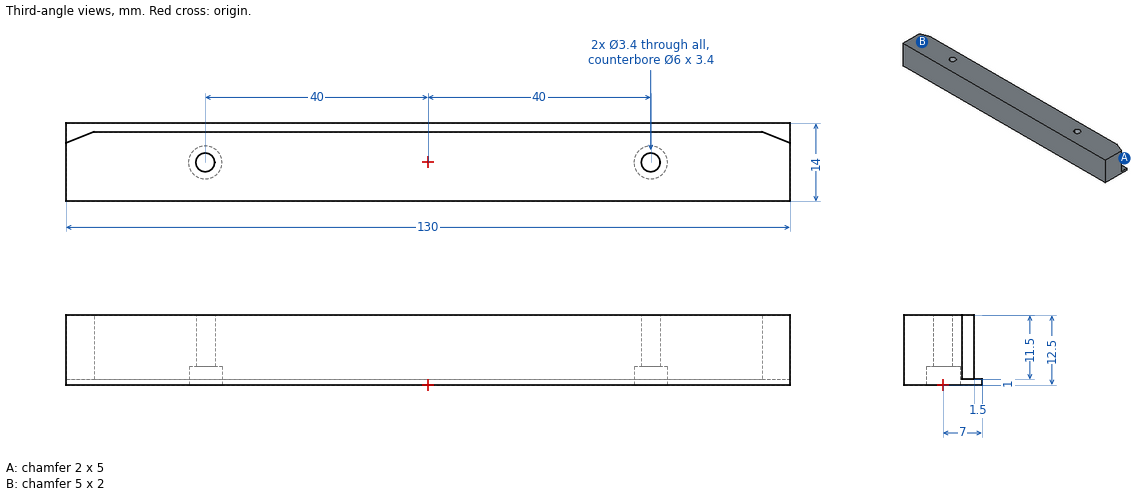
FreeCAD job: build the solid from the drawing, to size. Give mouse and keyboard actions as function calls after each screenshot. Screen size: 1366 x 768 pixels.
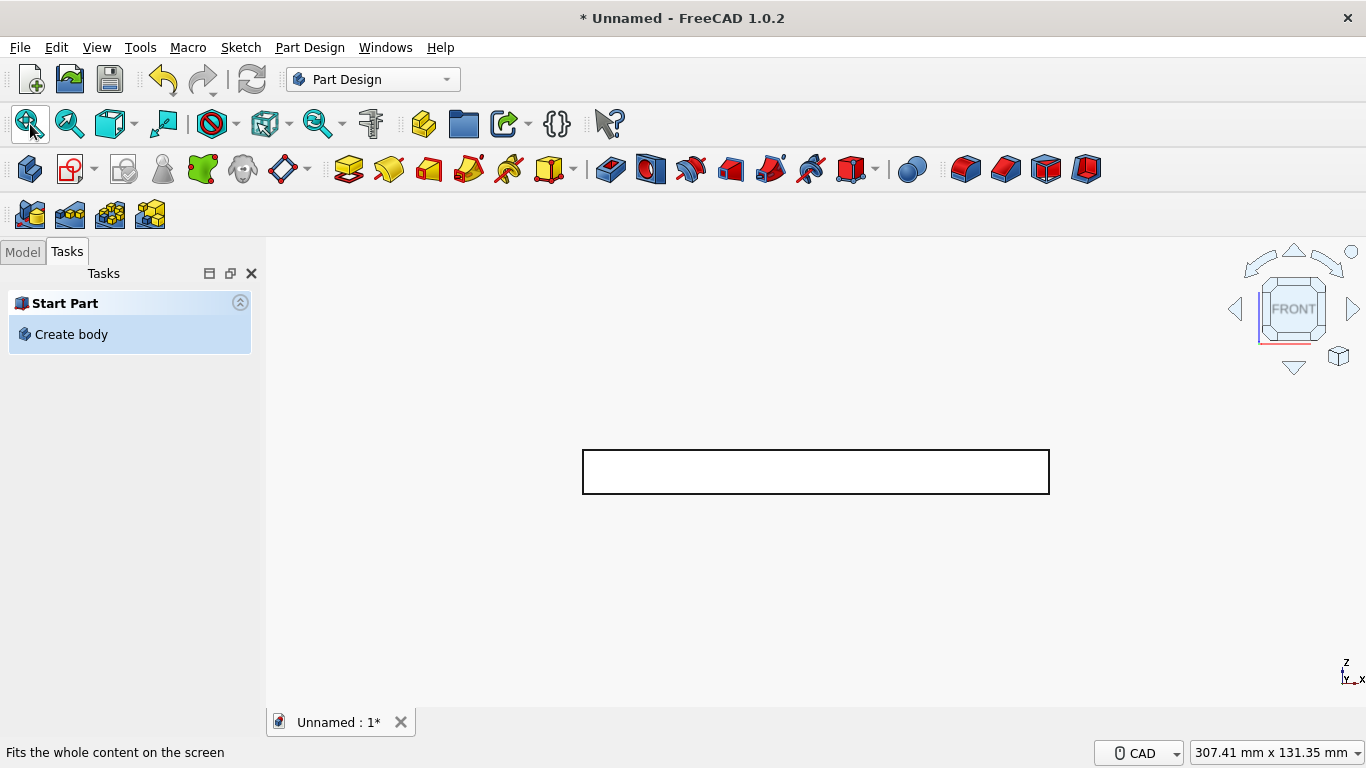
key(3)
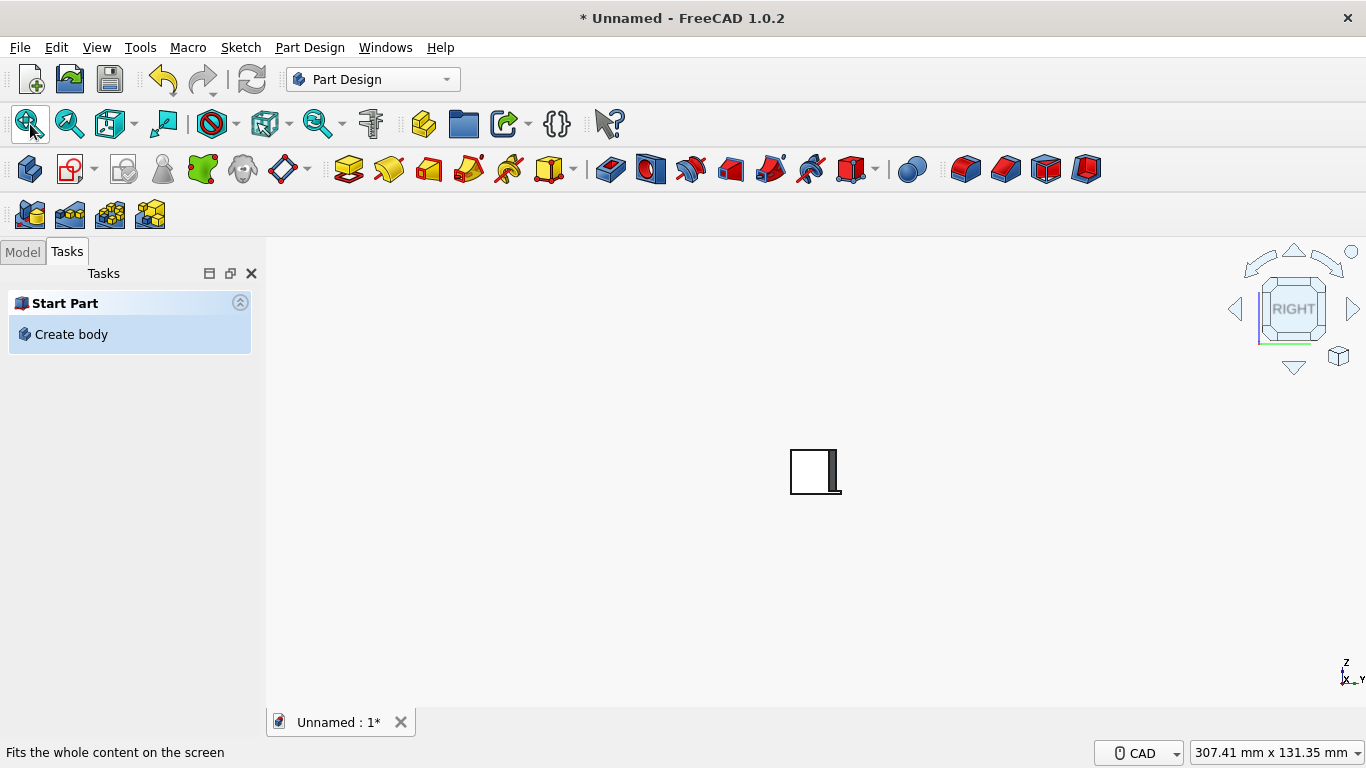
click(30, 124)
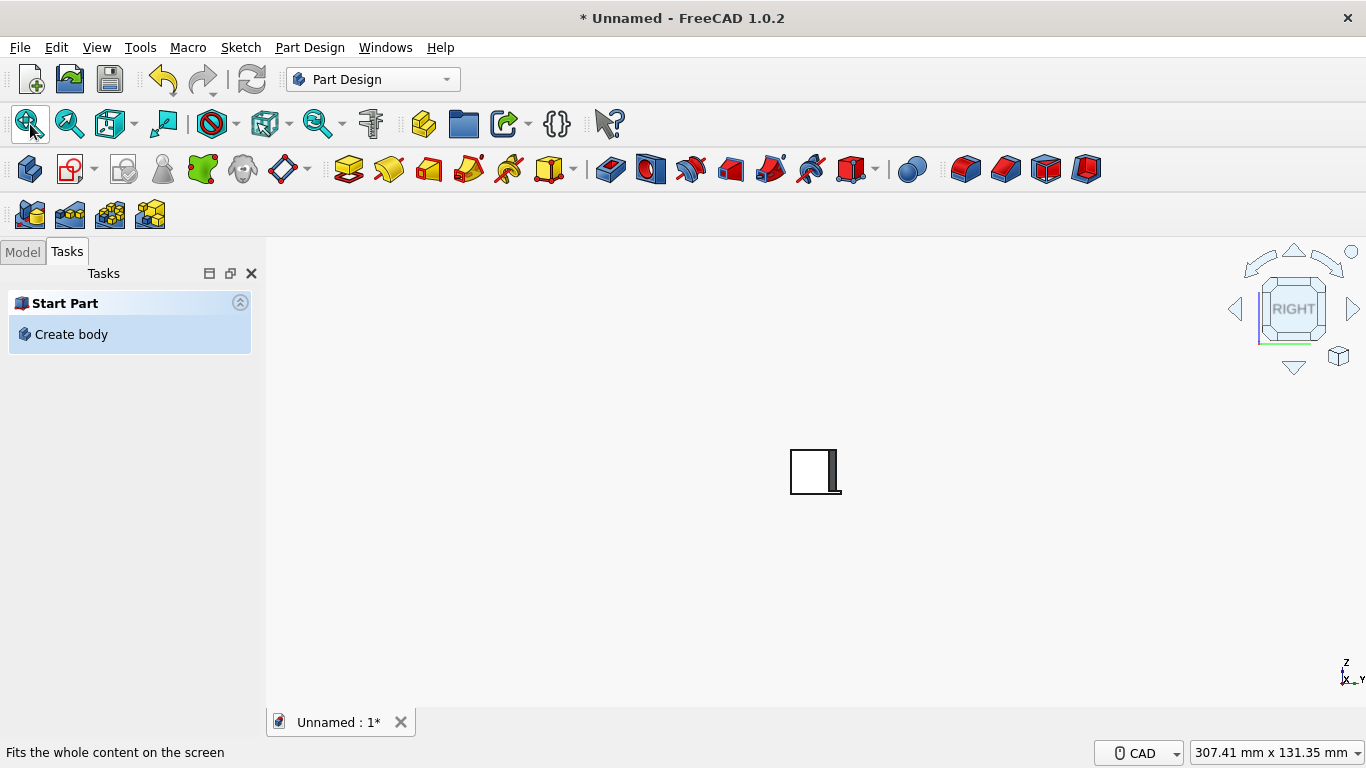
key(5)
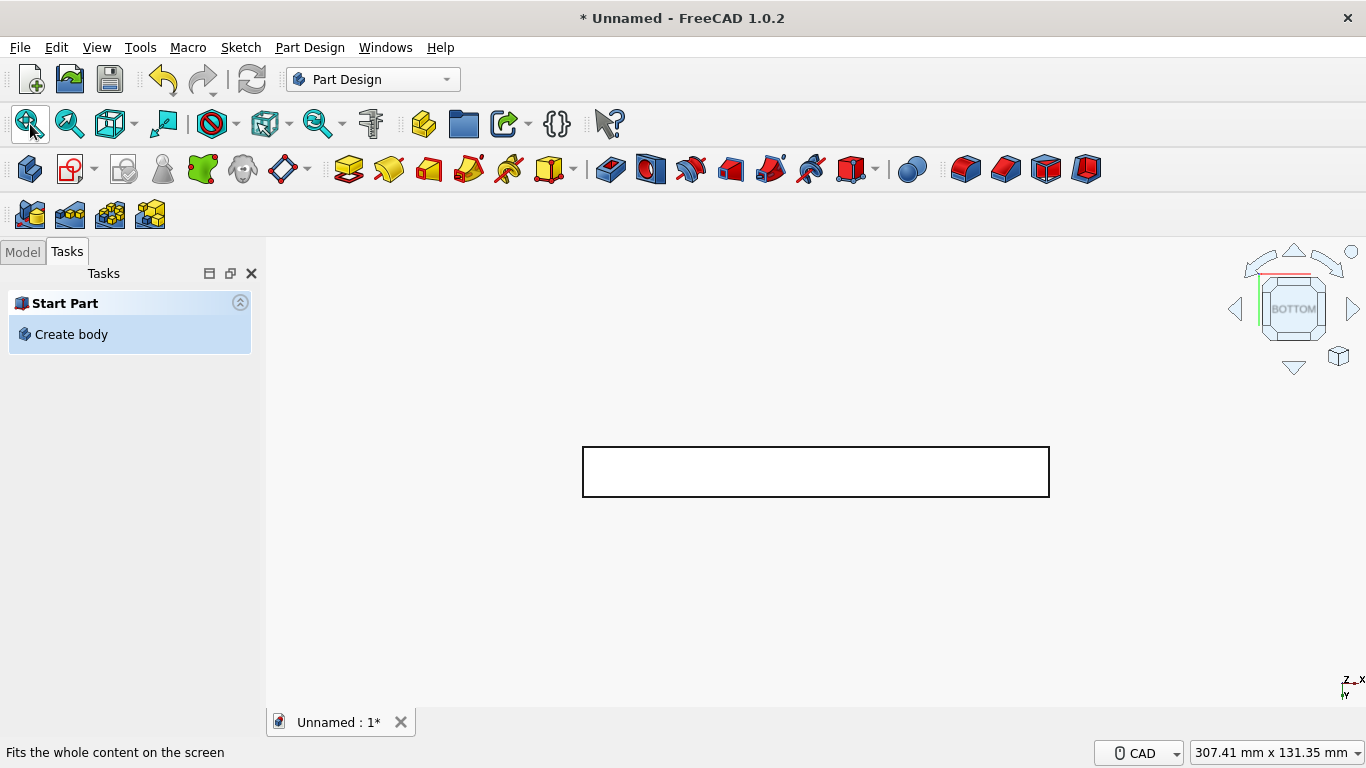
click(30, 124)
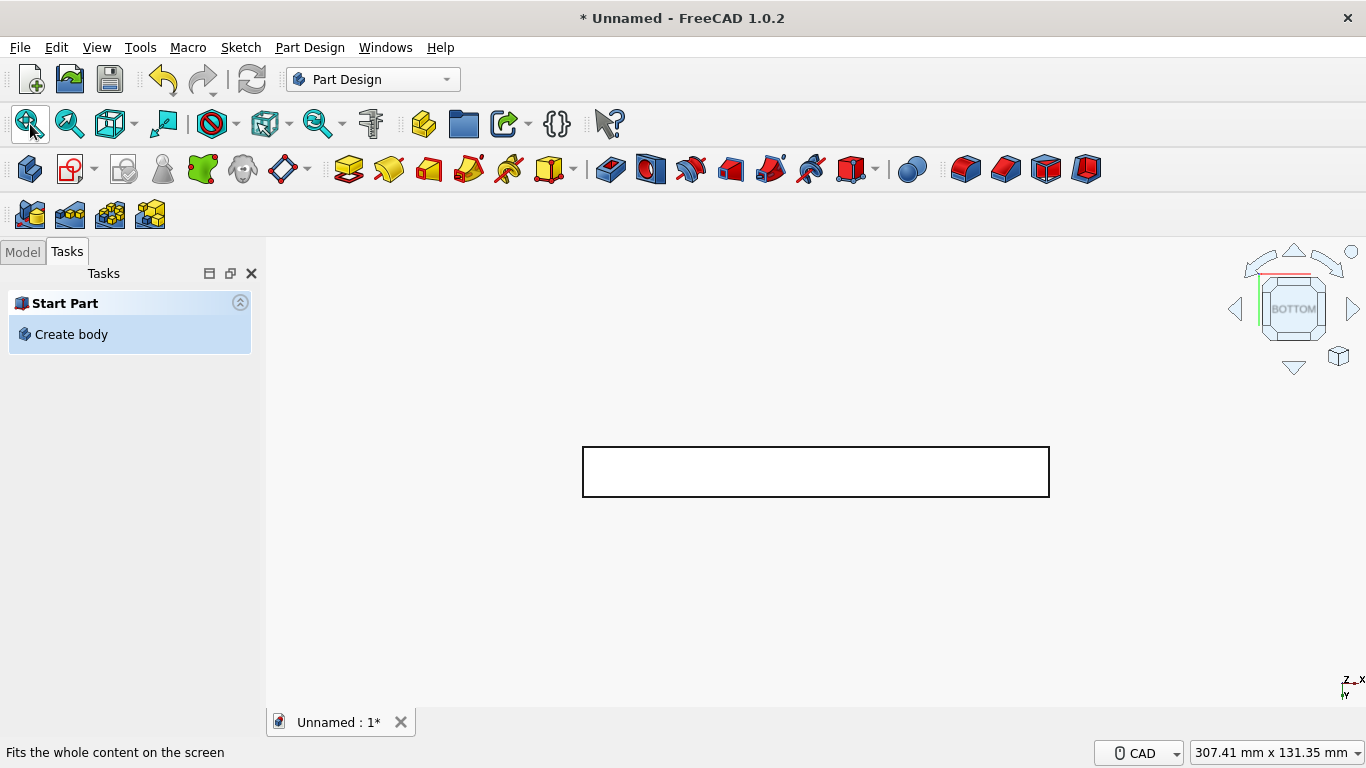
key(4)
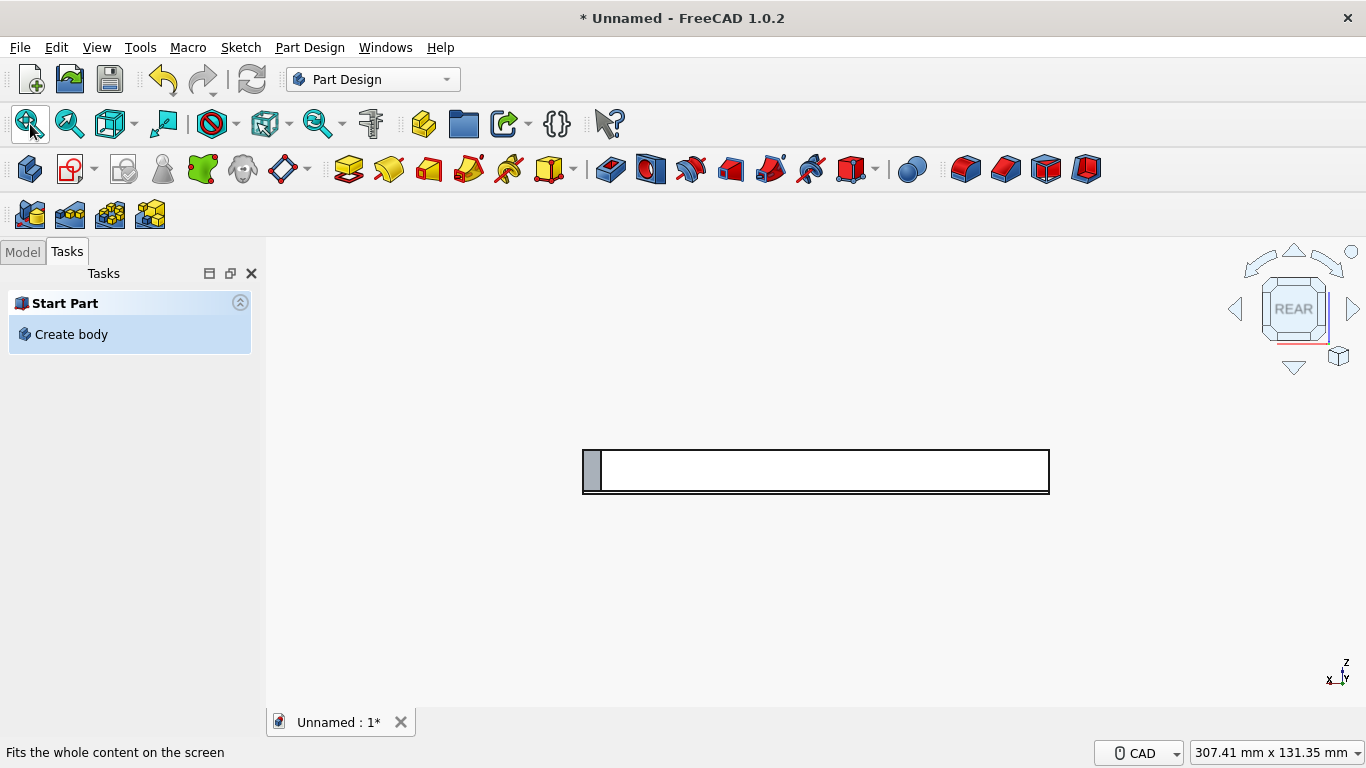
click(30, 124)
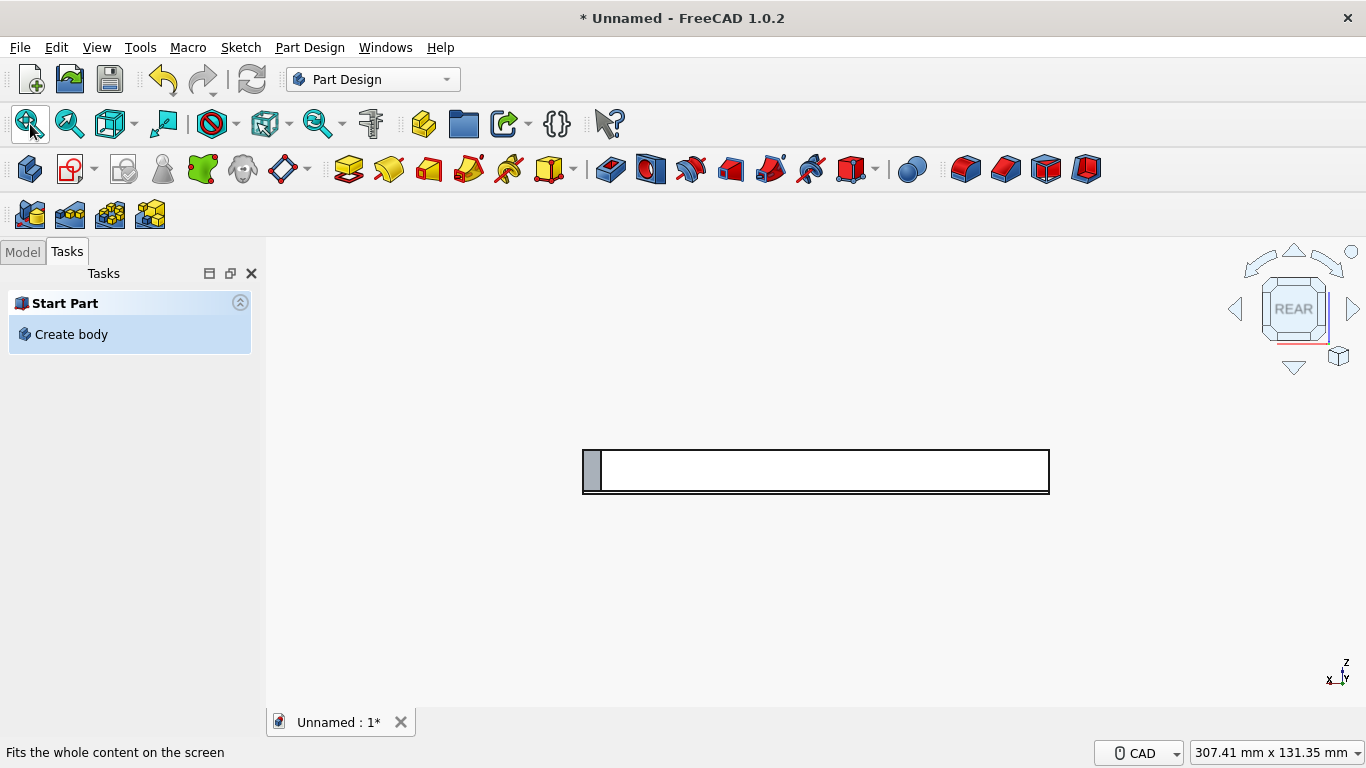
click(1049, 469)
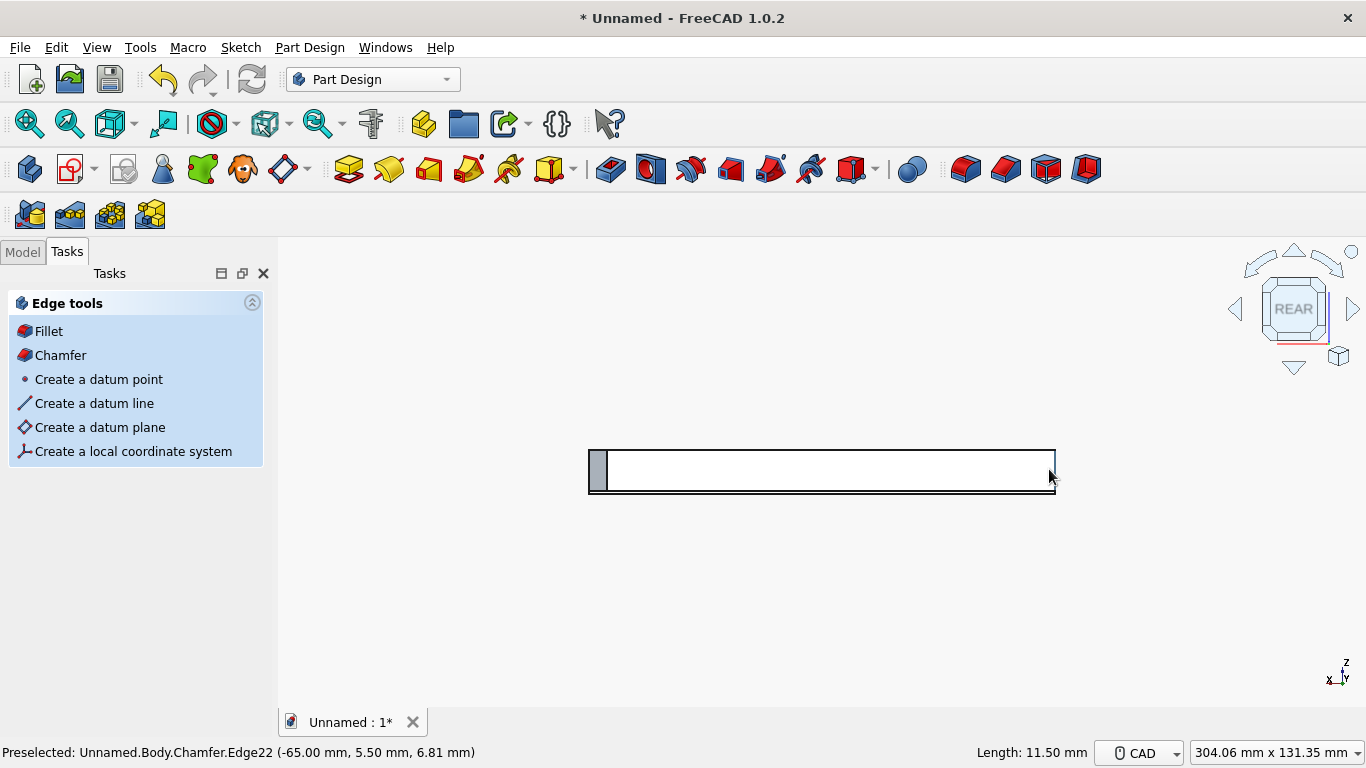
click(1006, 170)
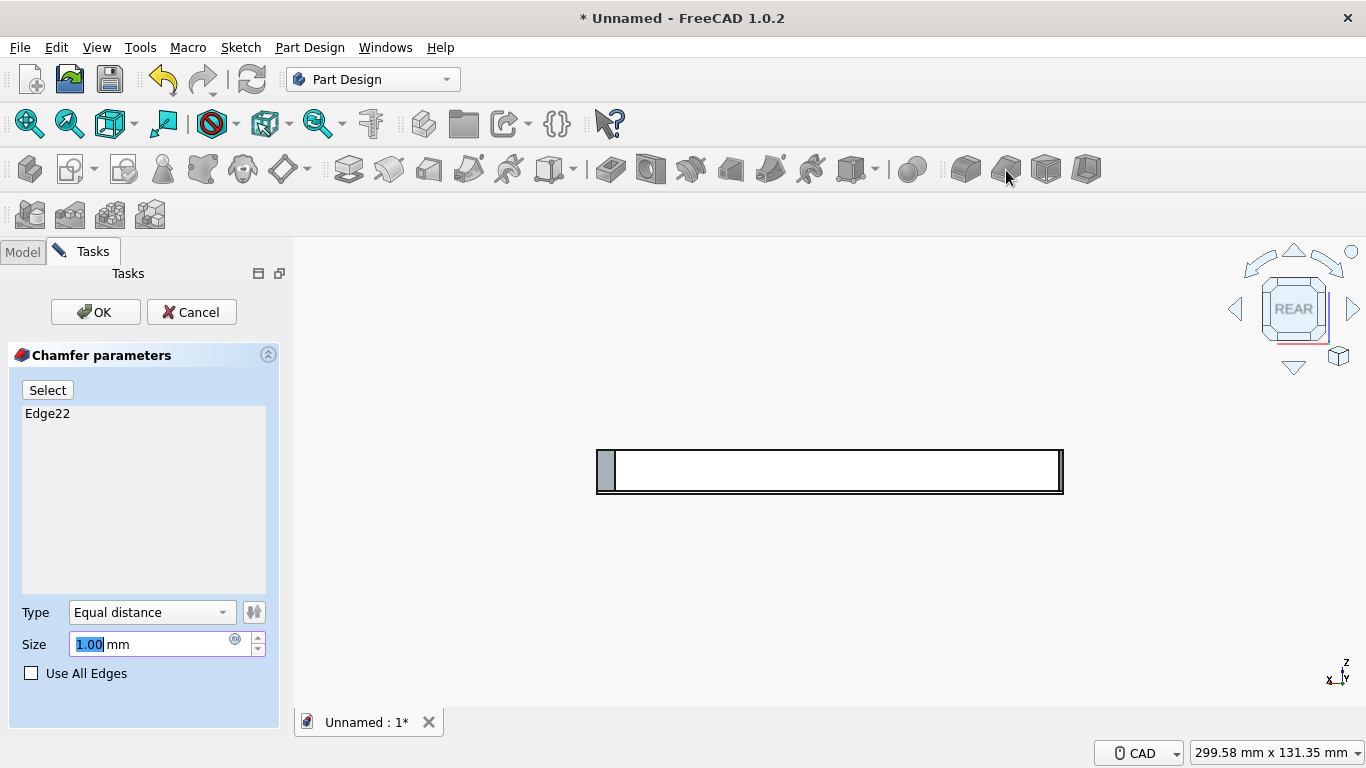
text(5)
key(Tab)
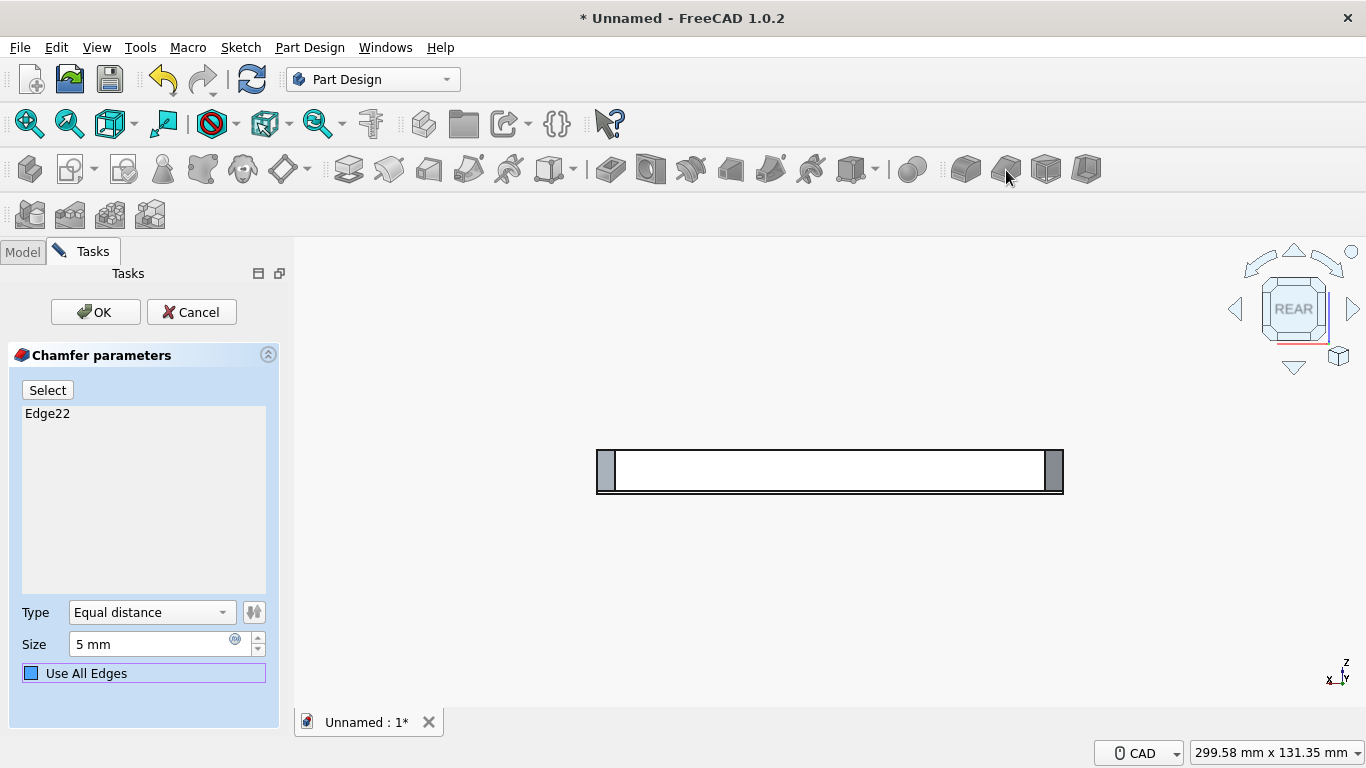
click(153, 612)